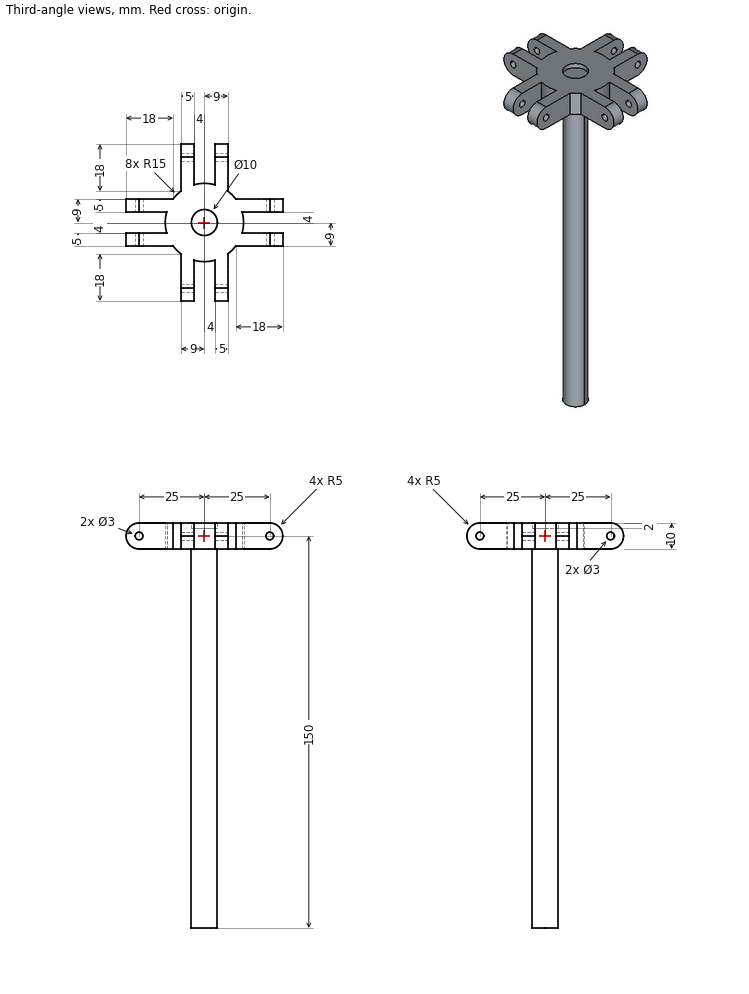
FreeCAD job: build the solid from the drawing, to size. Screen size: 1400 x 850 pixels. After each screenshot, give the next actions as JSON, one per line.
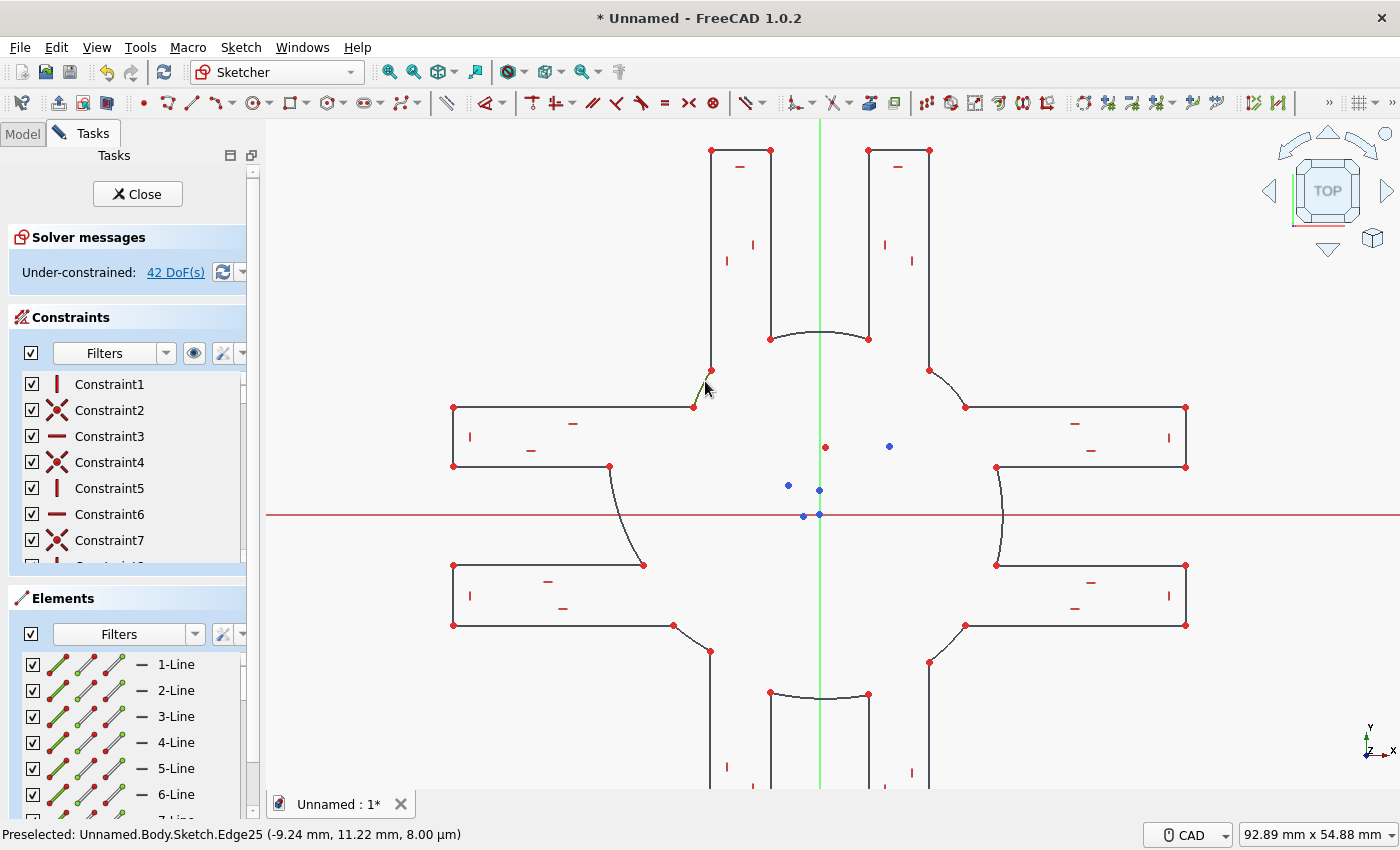
{"action": "left_click", "coordinate": [941, 652]}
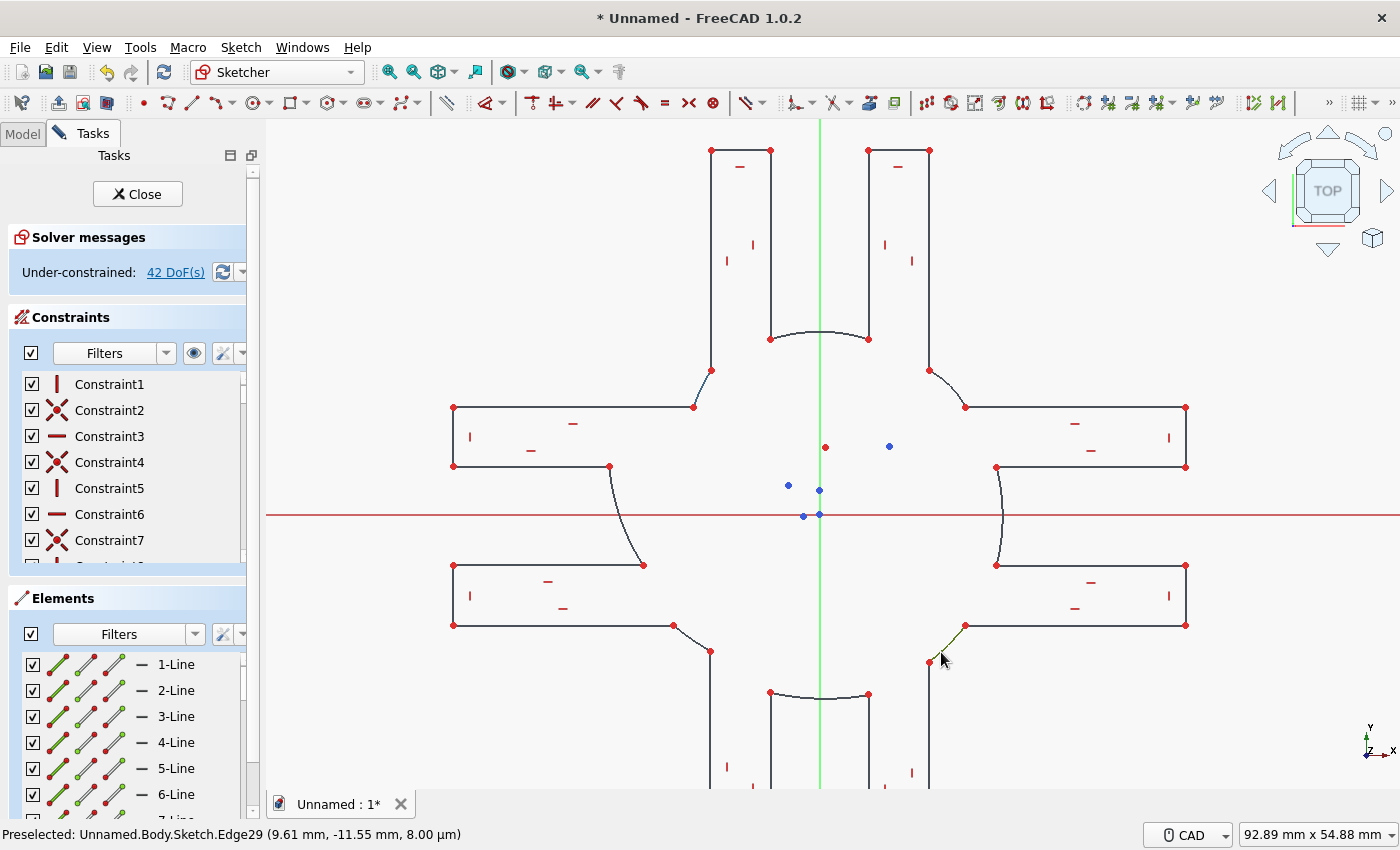
{"action": "left_click", "coordinate": [532, 104]}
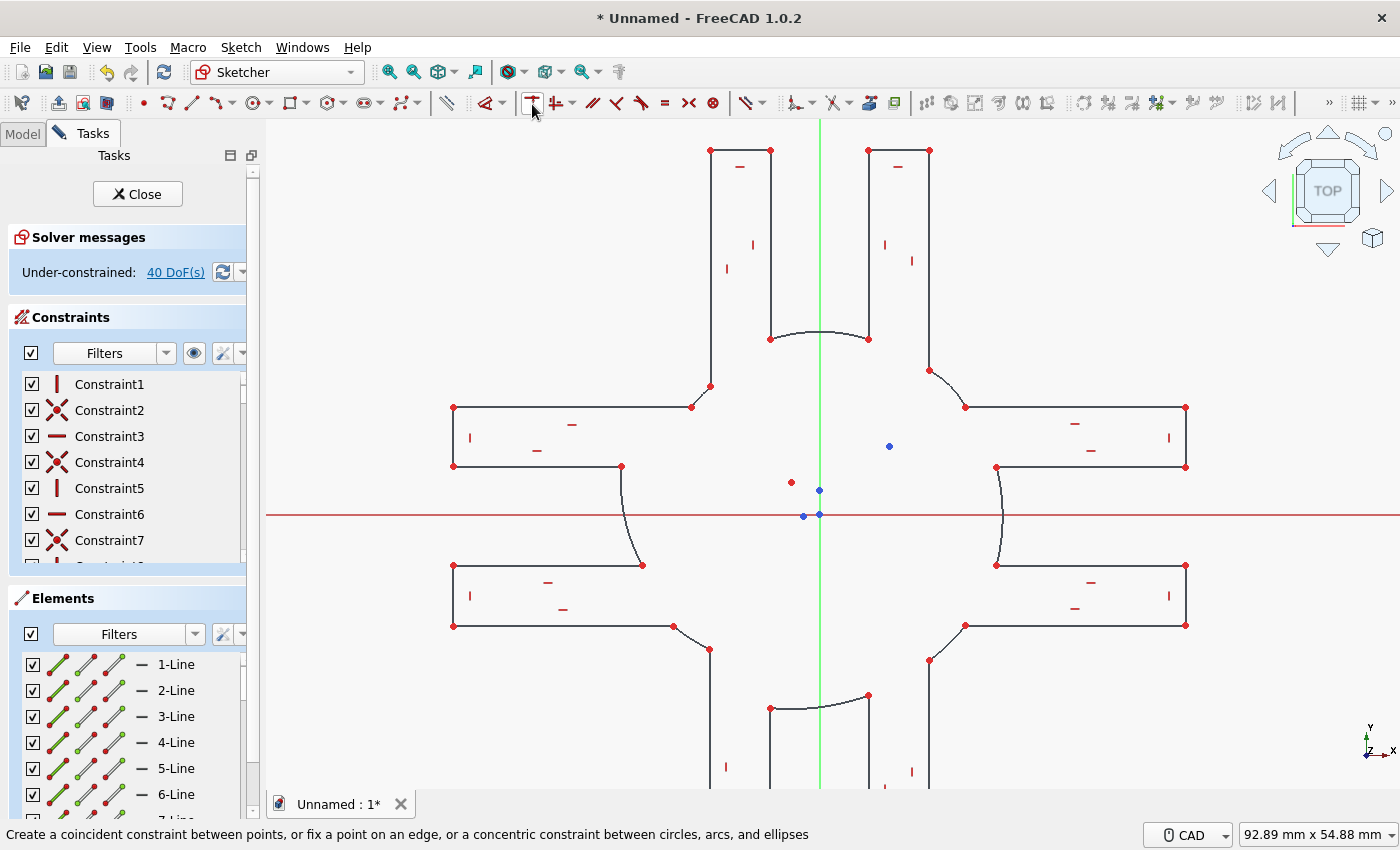
{"action": "left_click", "coordinate": [701, 396]}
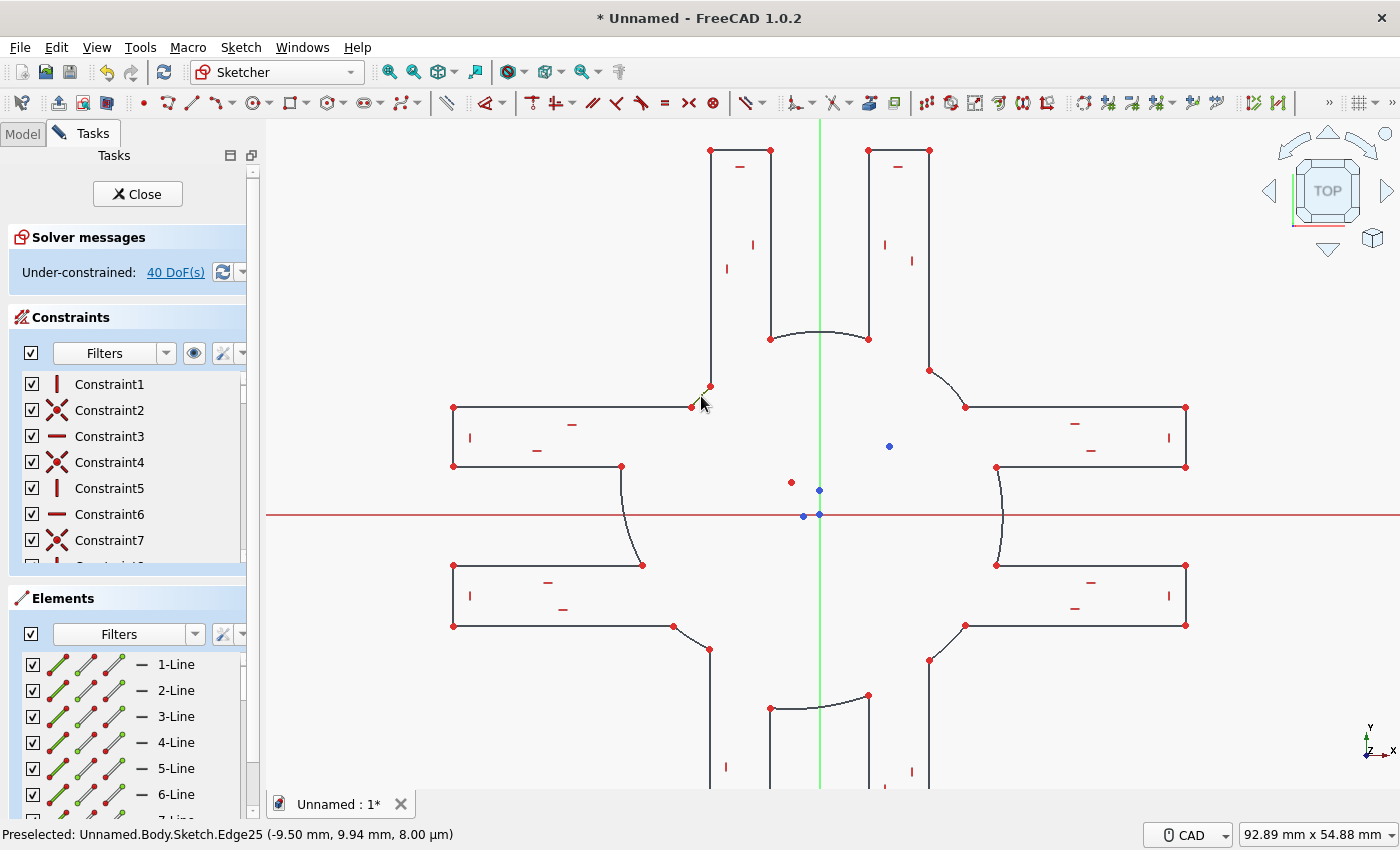
{"action": "left_click", "coordinate": [1002, 536]}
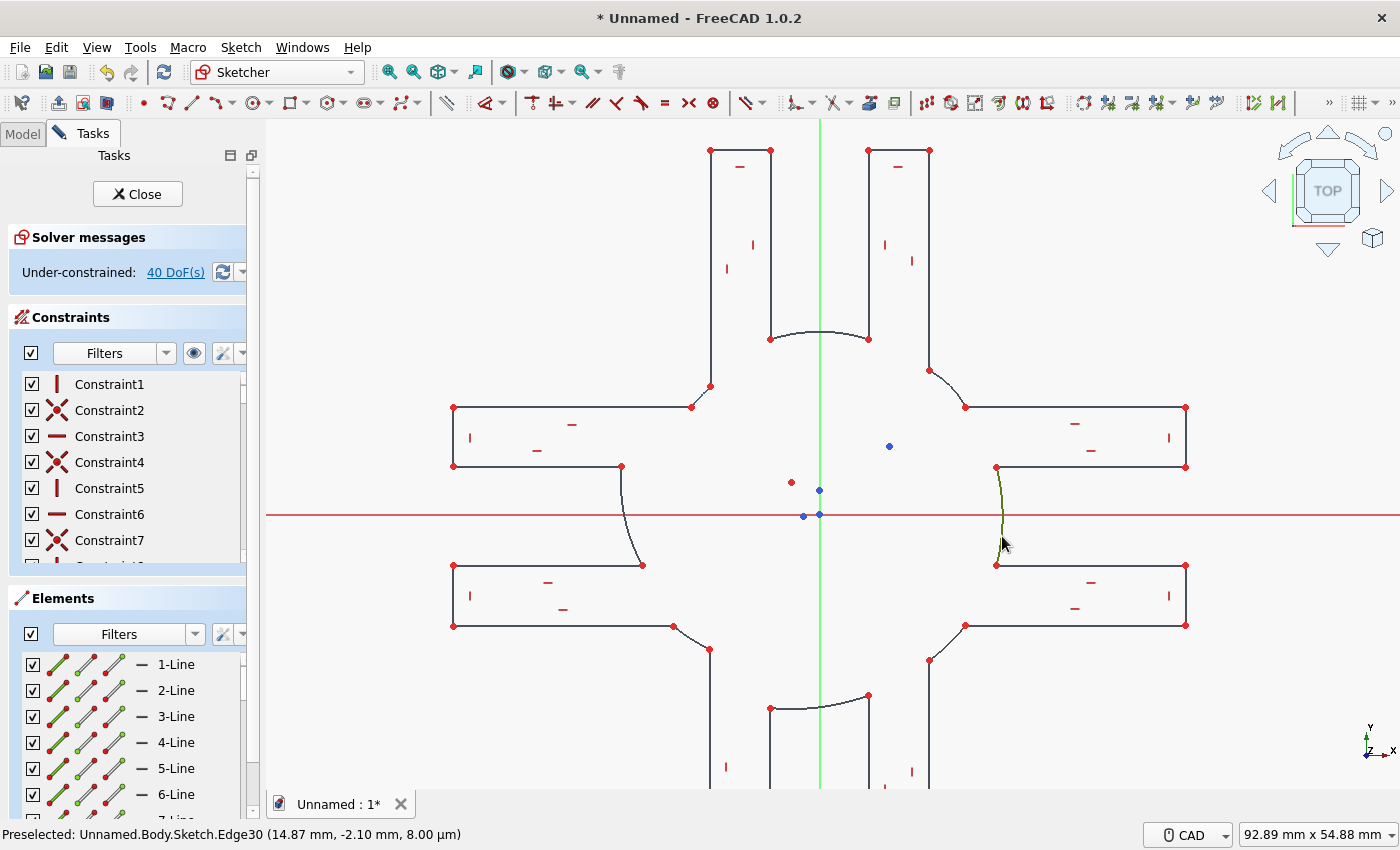
{"action": "left_click", "coordinate": [532, 104]}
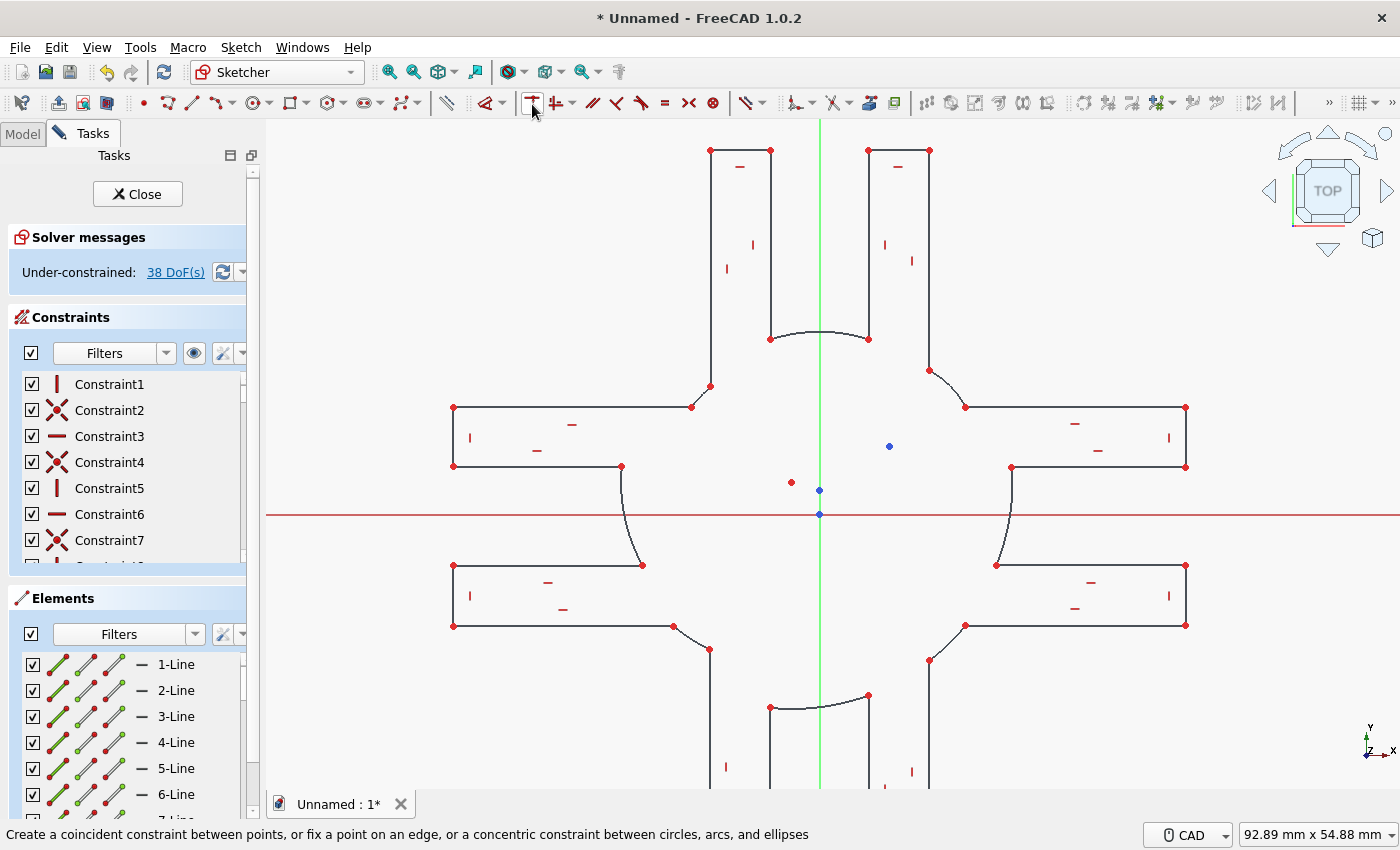
{"action": "left_click", "coordinate": [701, 396]}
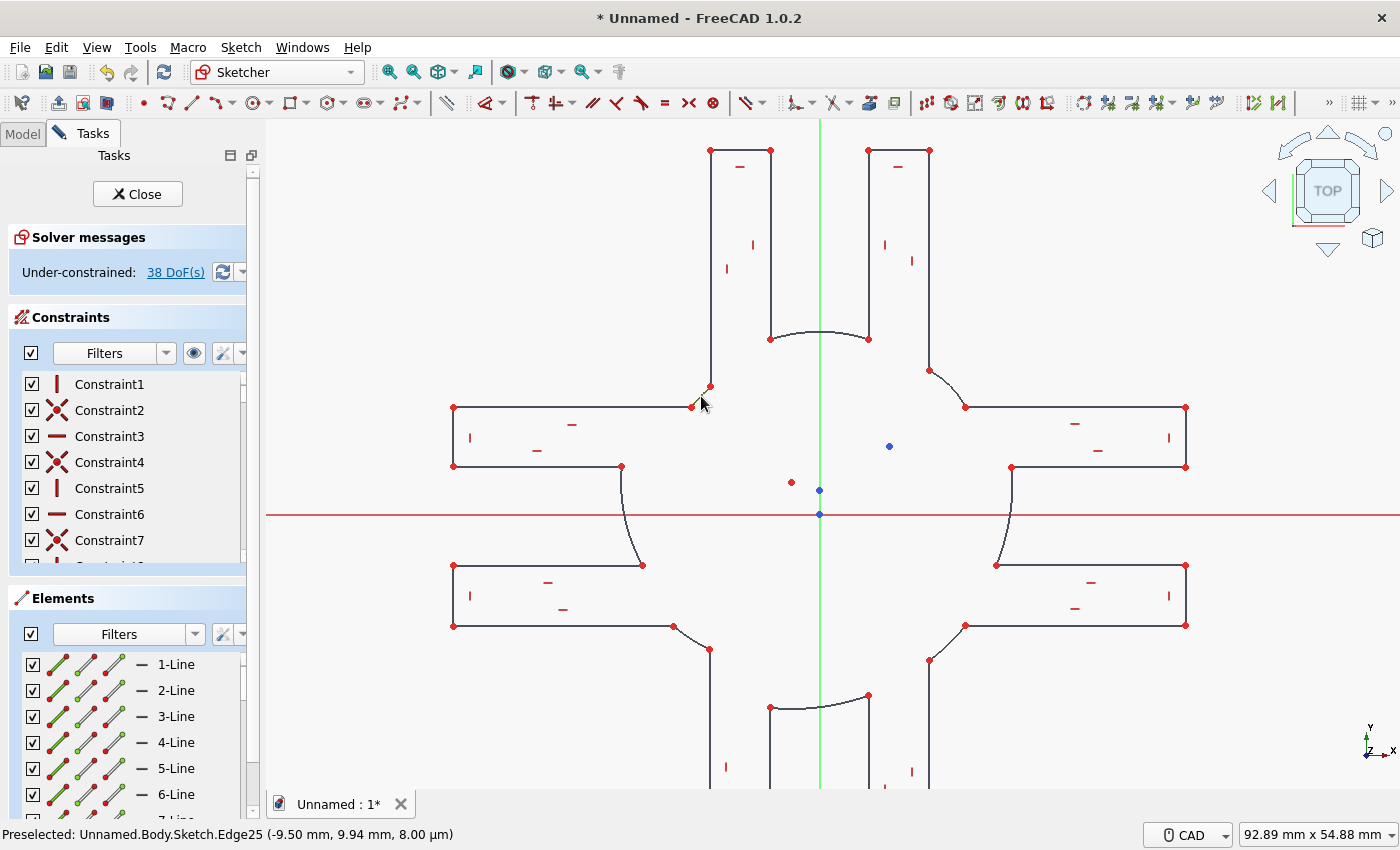
{"action": "left_click", "coordinate": [957, 394]}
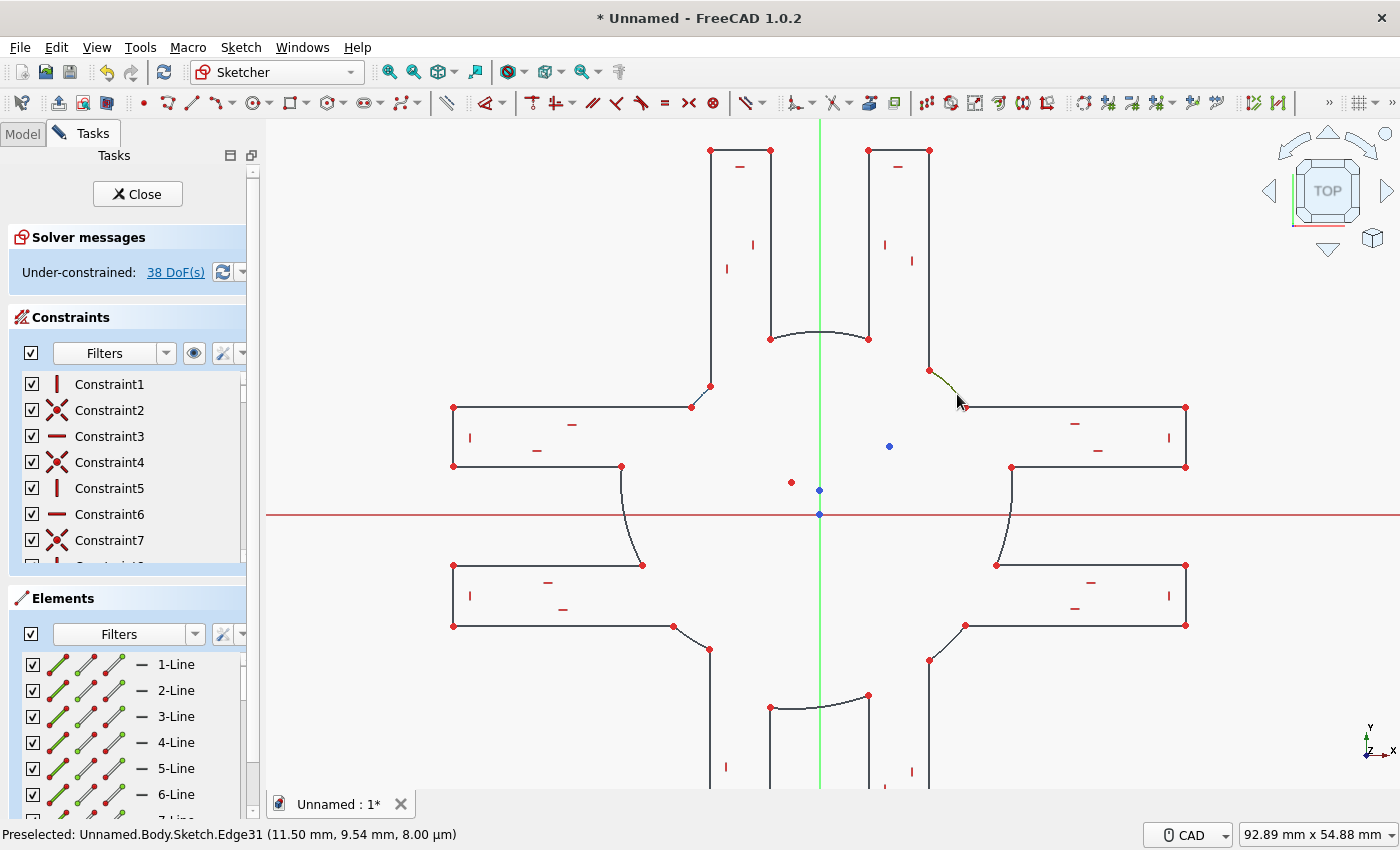
{"action": "key", "text": "c"}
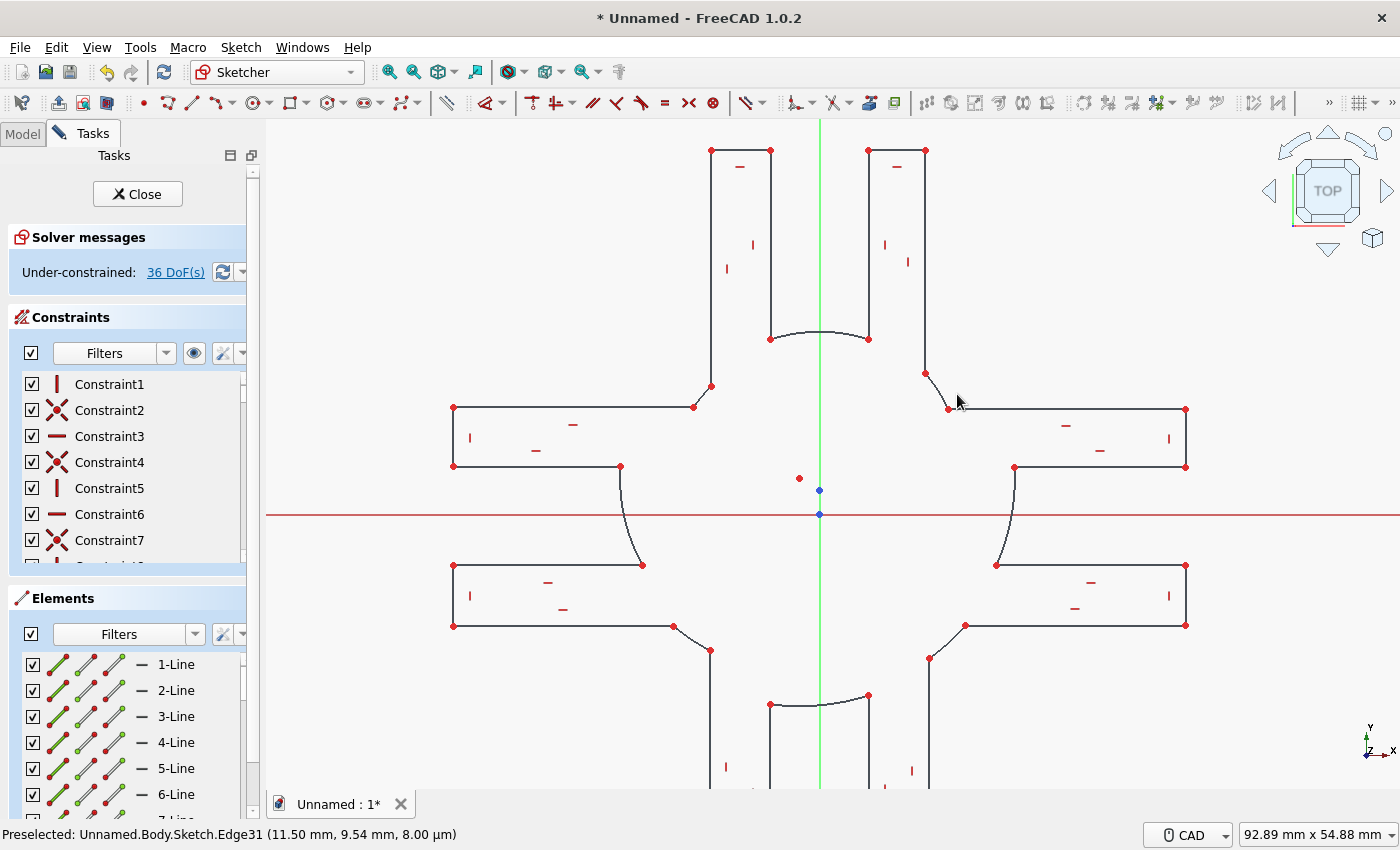
{"action": "left_click", "coordinate": [702, 397]}